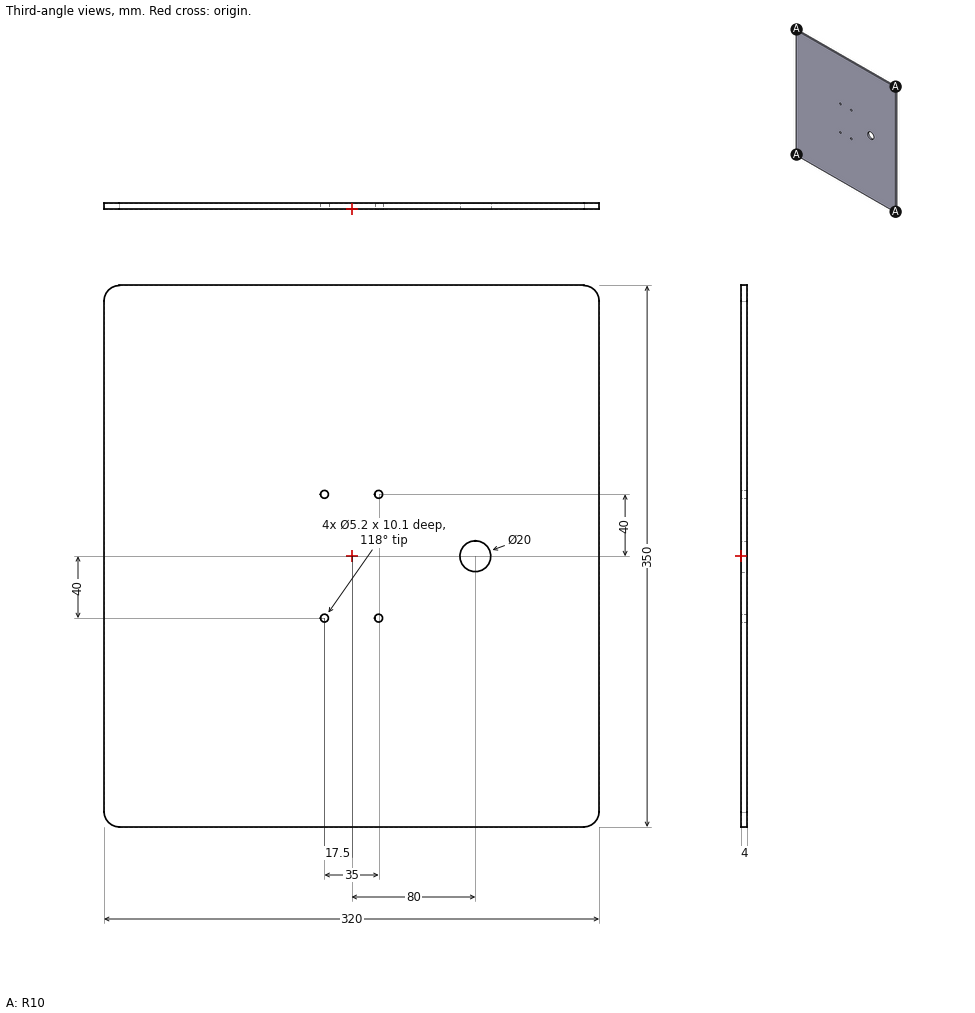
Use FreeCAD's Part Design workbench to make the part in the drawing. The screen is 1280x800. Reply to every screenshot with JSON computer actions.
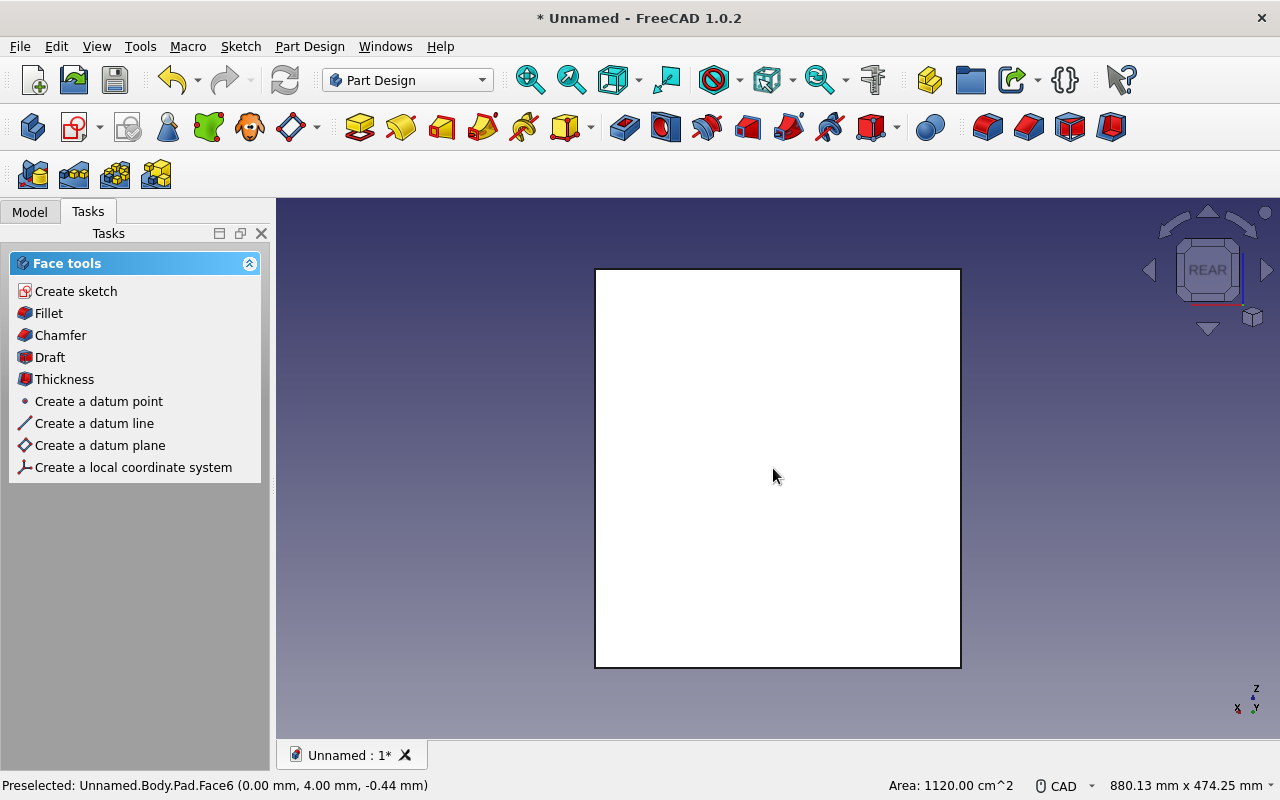
{"action": "left_click", "coordinate": [74, 128]}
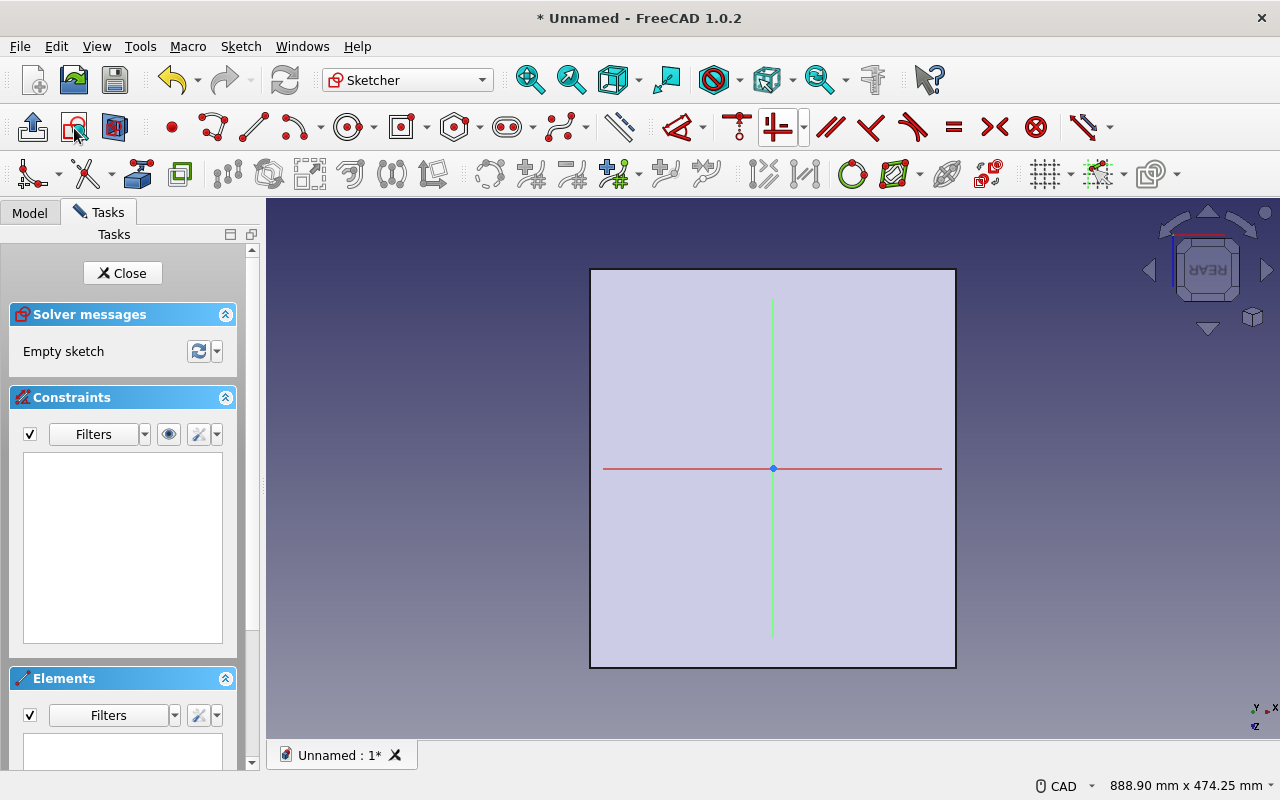
{"action": "scroll", "coordinate": [803, 468], "scroll_direction": "up", "scroll_amount": 6}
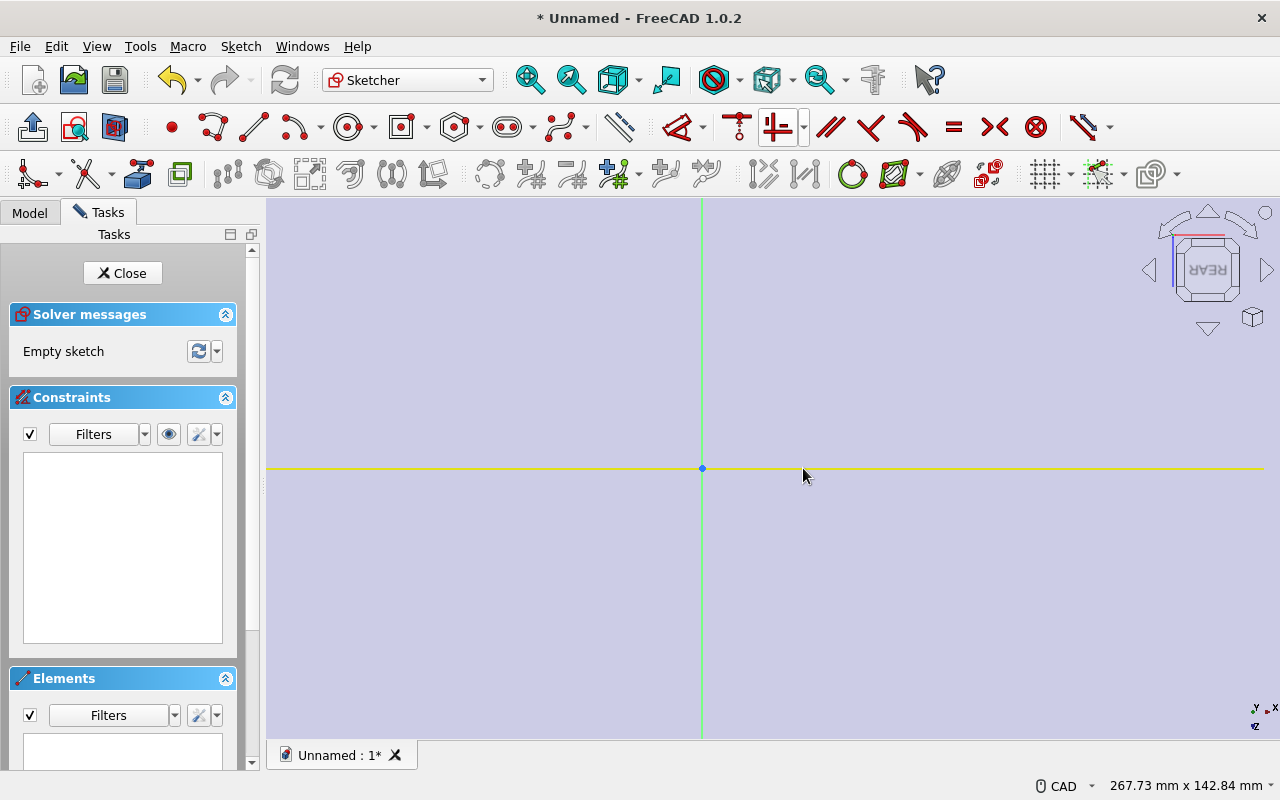
{"action": "left_click", "coordinate": [348, 128]}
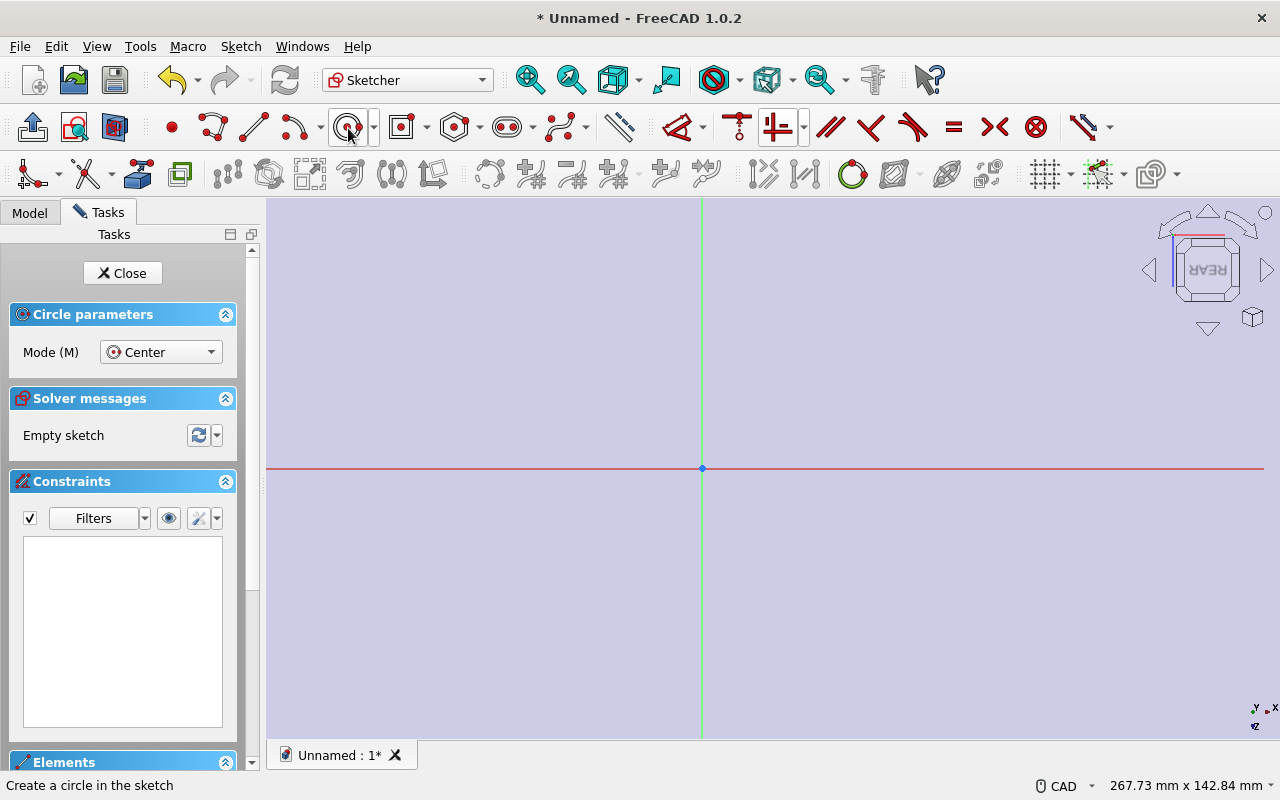
{"action": "scroll", "coordinate": [636, 317], "scroll_direction": "up", "scroll_amount": 5}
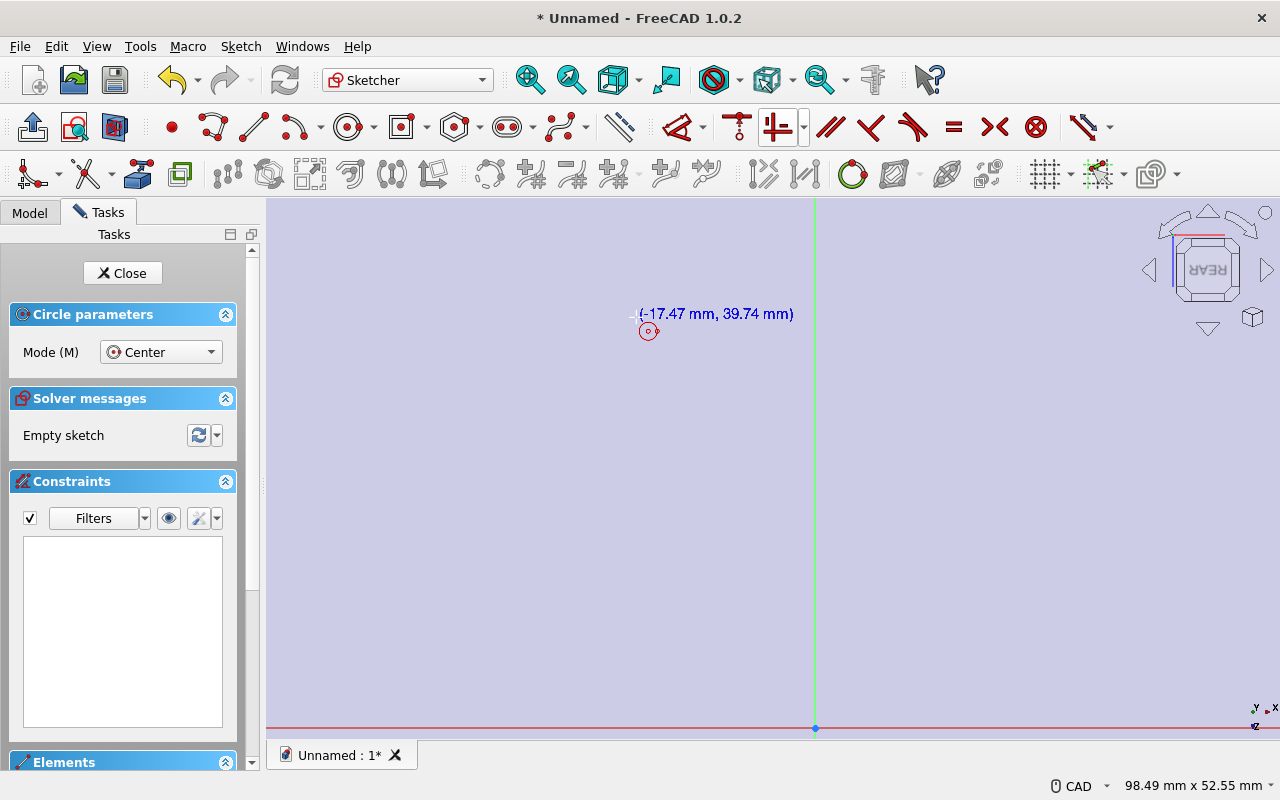
{"action": "left_click", "coordinate": [635, 317]}
{"action": "left_click", "coordinate": [654, 298]}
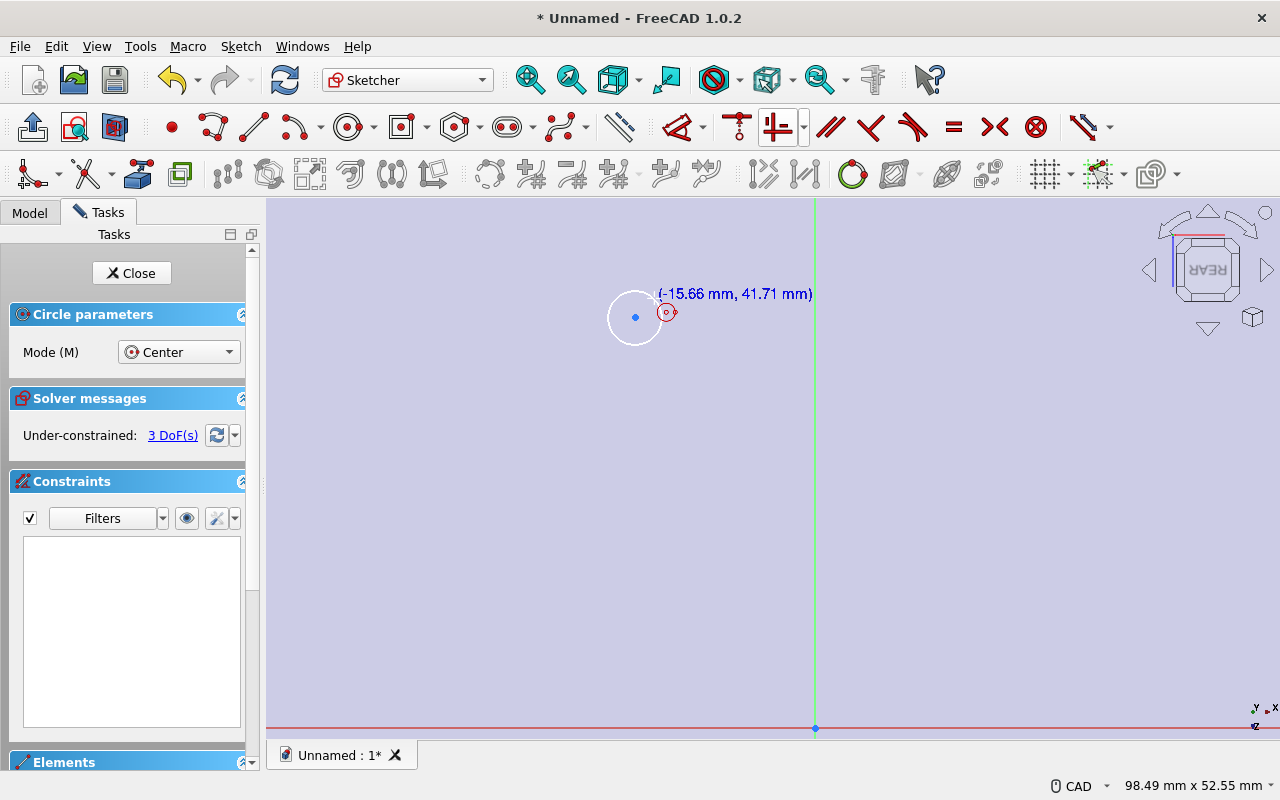
{"action": "scroll", "coordinate": [640, 317], "scroll_direction": "down", "scroll_amount": 5}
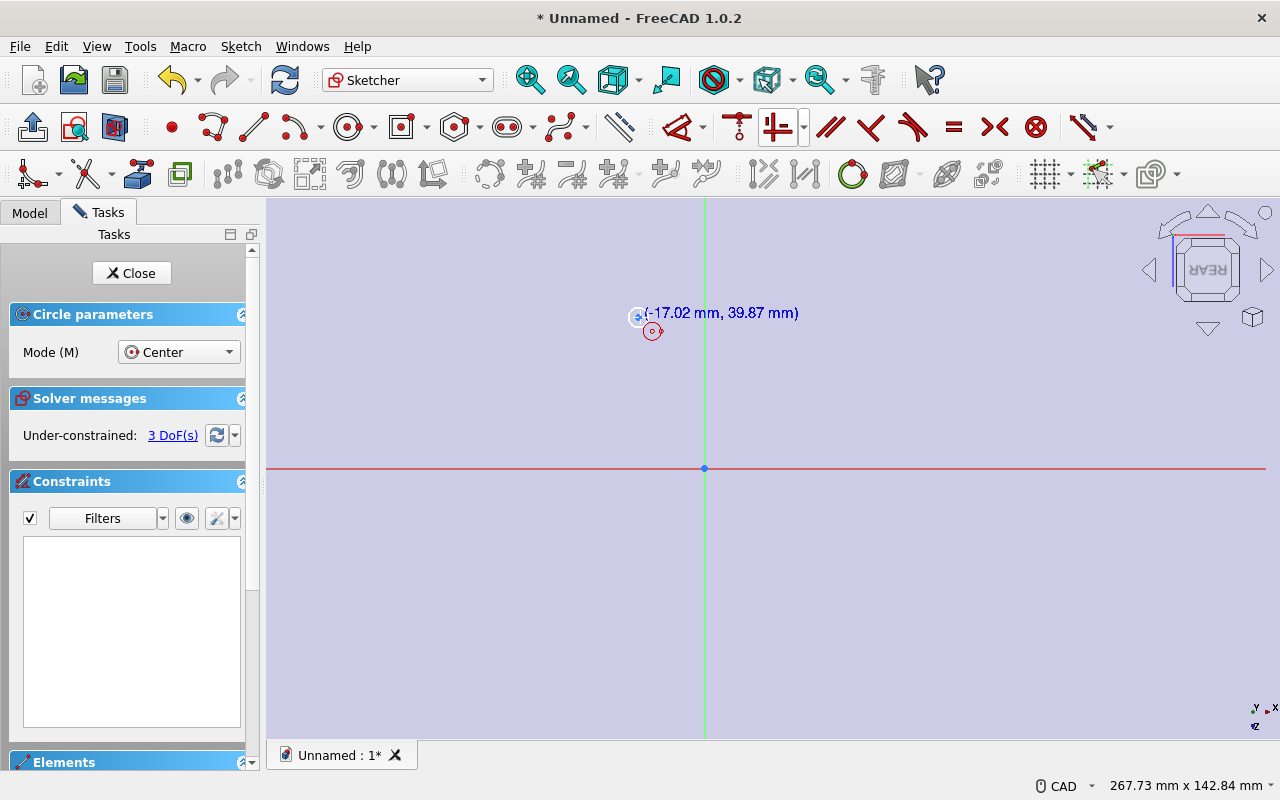
{"action": "scroll", "coordinate": [771, 620], "scroll_direction": "up", "scroll_amount": 5}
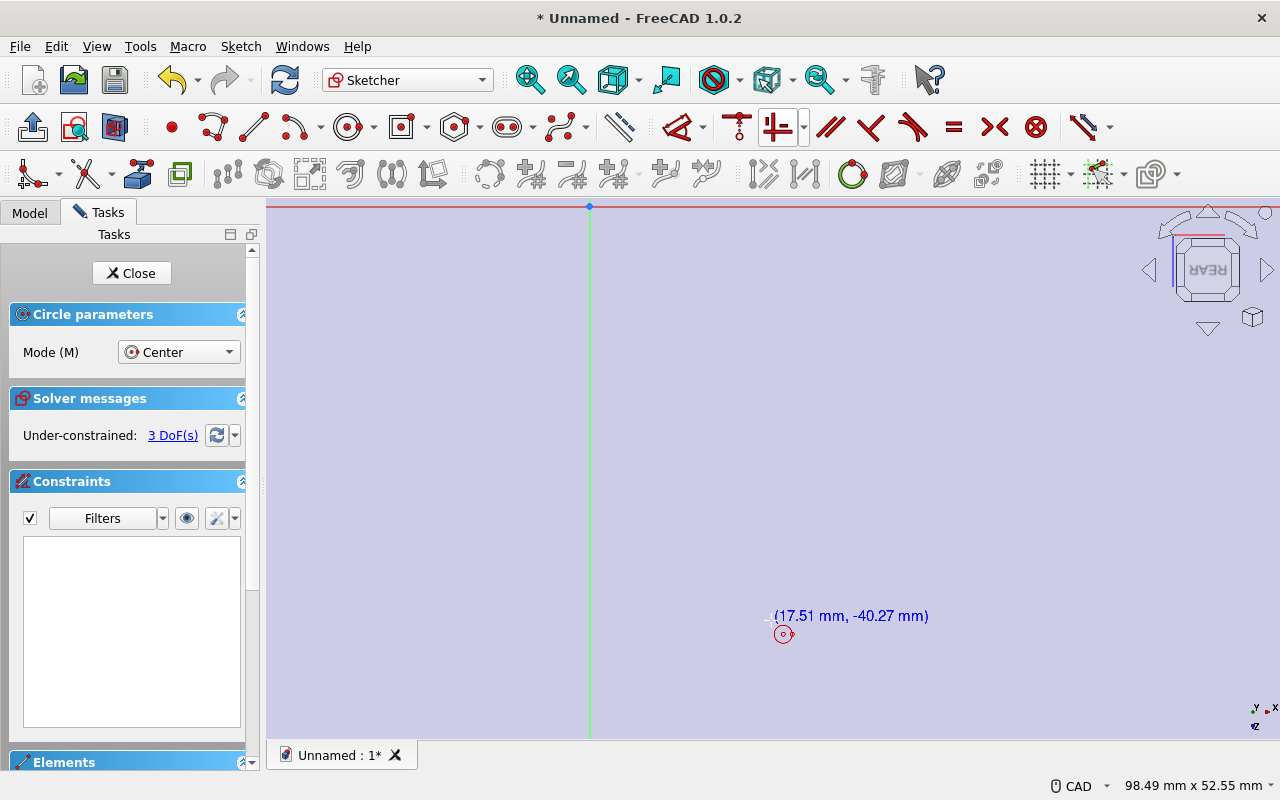
{"action": "left_click", "coordinate": [770, 619]}
{"action": "left_click", "coordinate": [789, 600]}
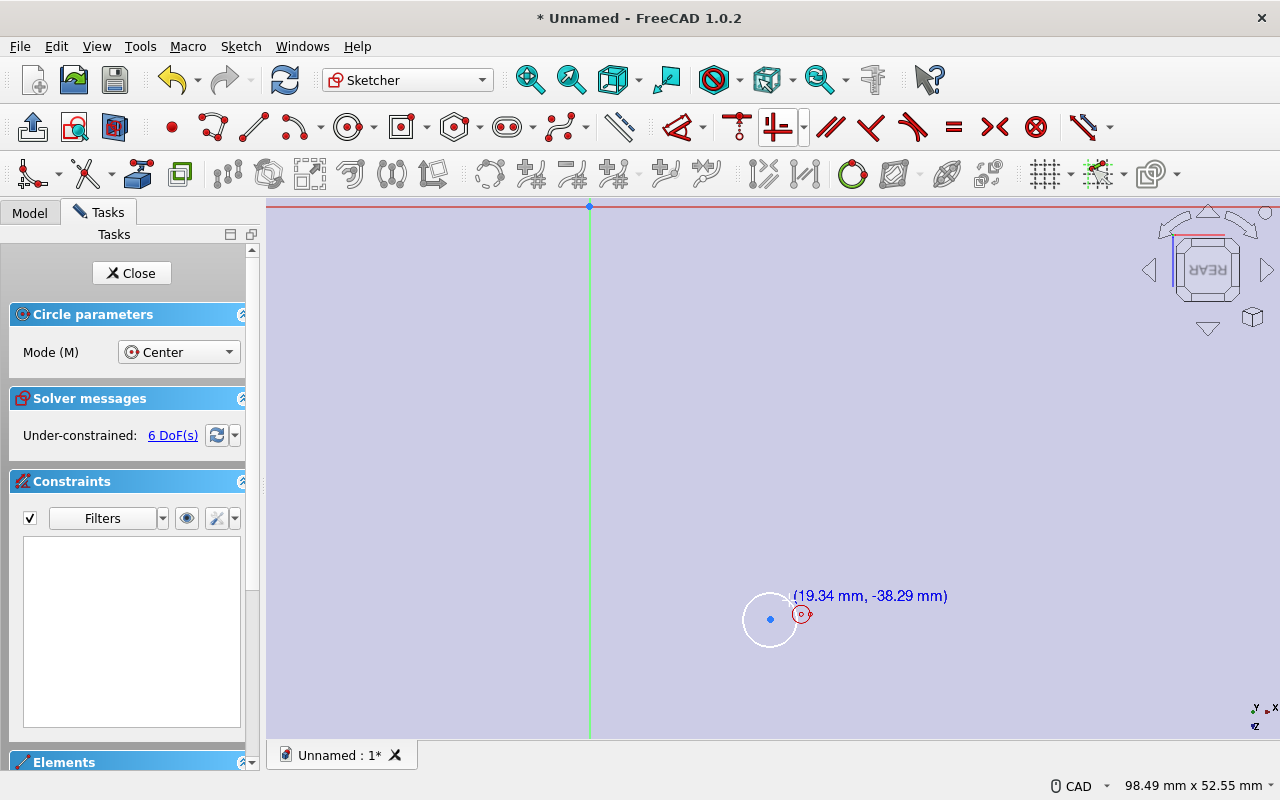
{"action": "left_click", "coordinate": [410, 619]}
{"action": "left_click", "coordinate": [429, 600]}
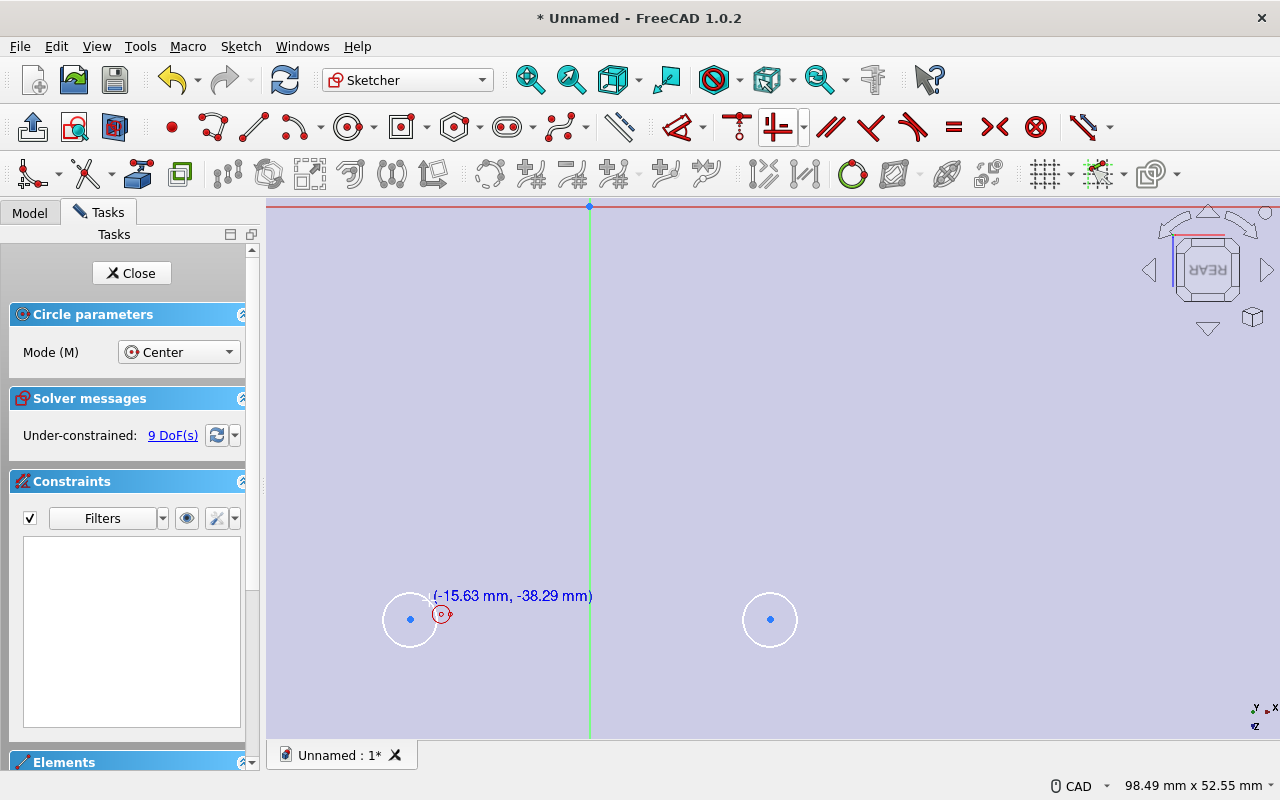
{"action": "scroll", "coordinate": [771, 621], "scroll_direction": "down", "scroll_amount": 5}